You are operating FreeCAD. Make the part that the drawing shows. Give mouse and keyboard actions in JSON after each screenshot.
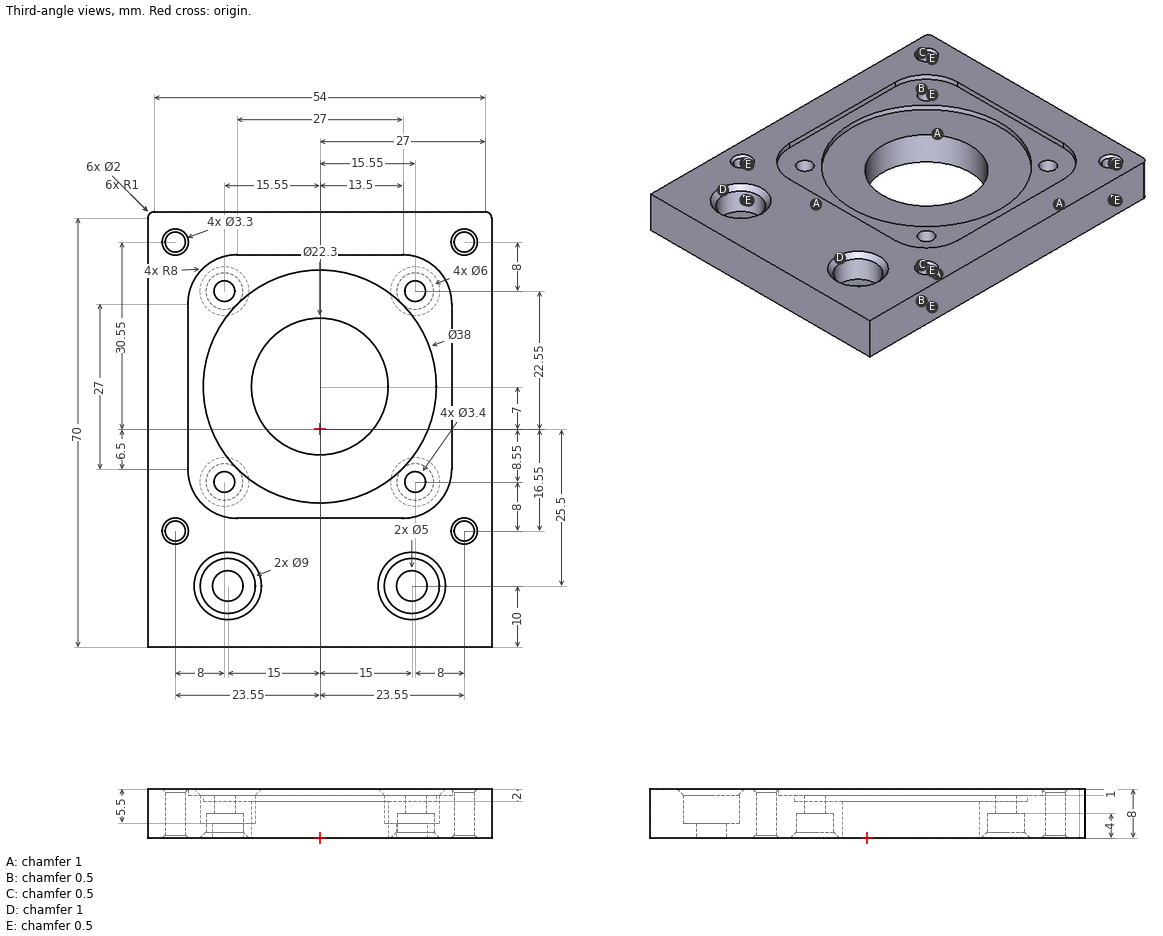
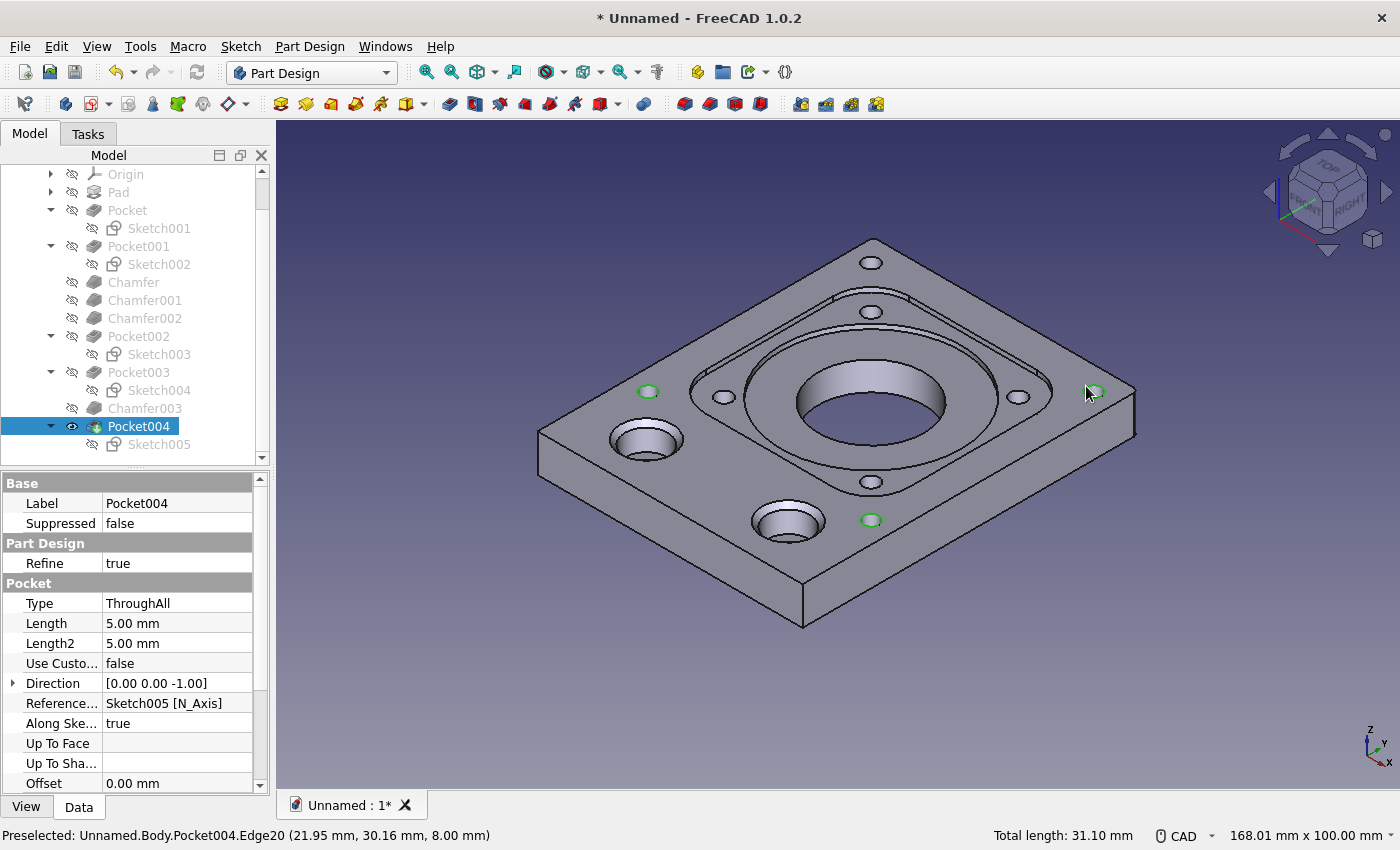
{"action": "left_click", "coordinate": [863, 258], "text": "ctrl"}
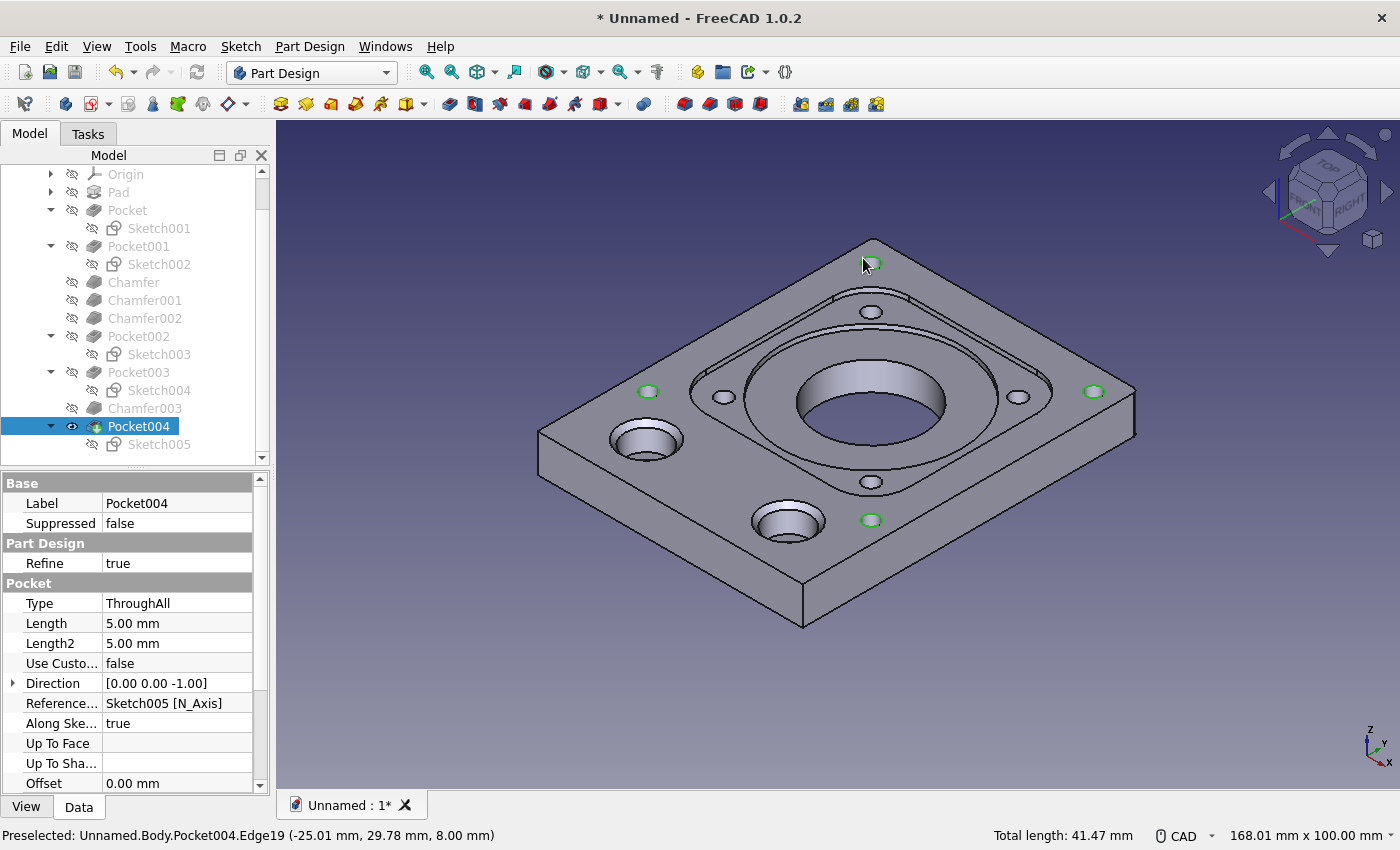
{"action": "key", "text": "2"}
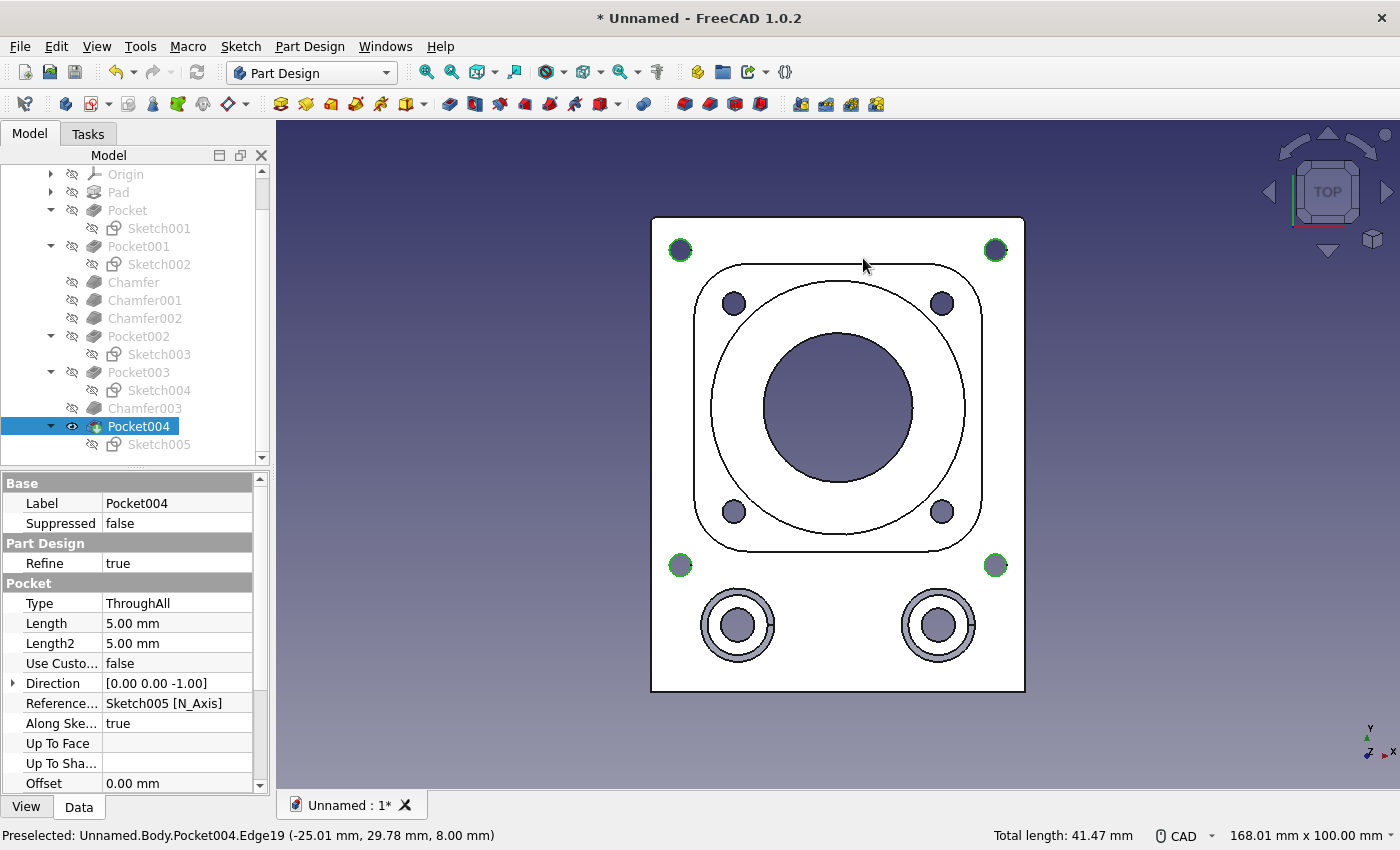
{"action": "key", "text": "0"}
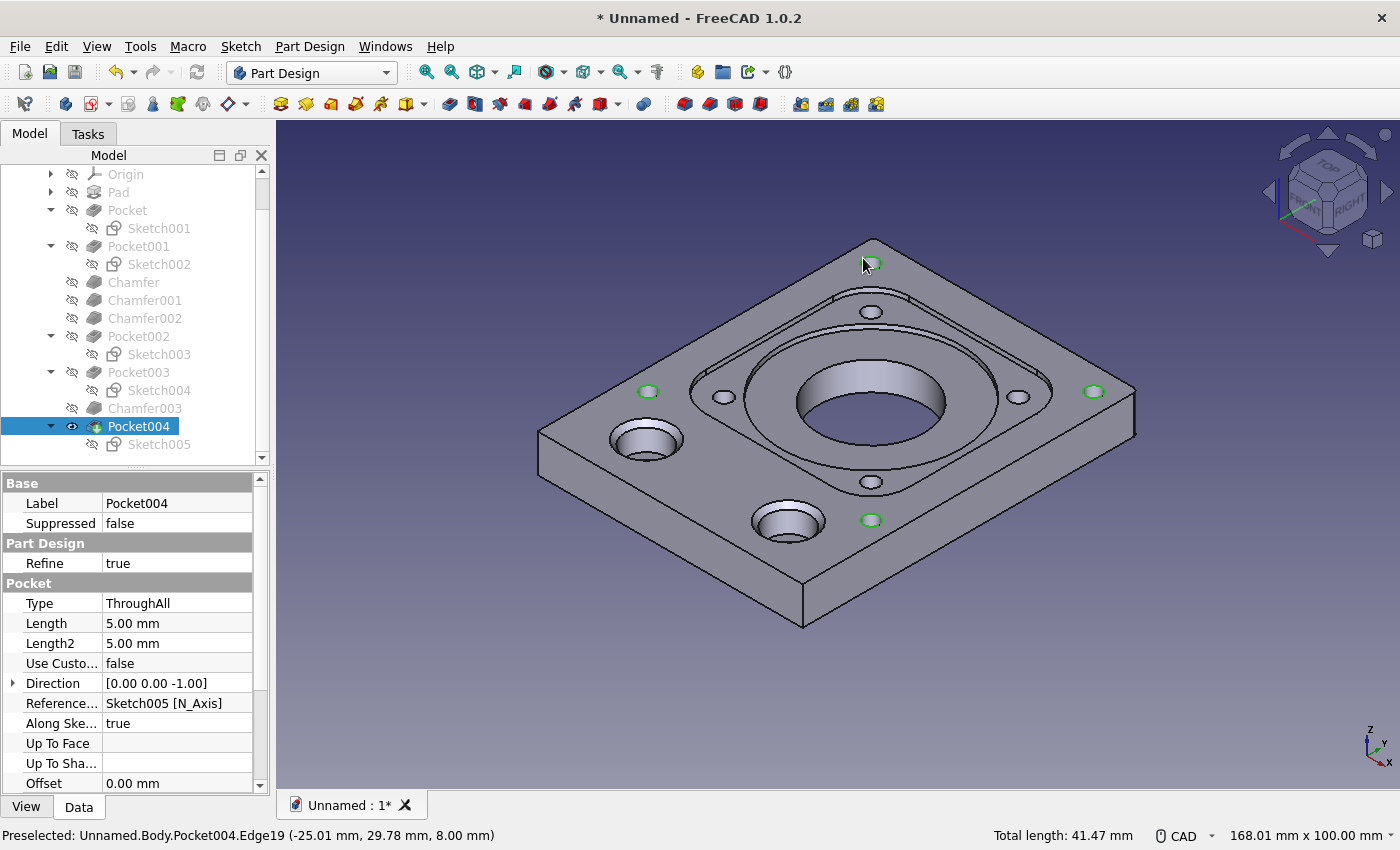
{"action": "key", "text": "1"}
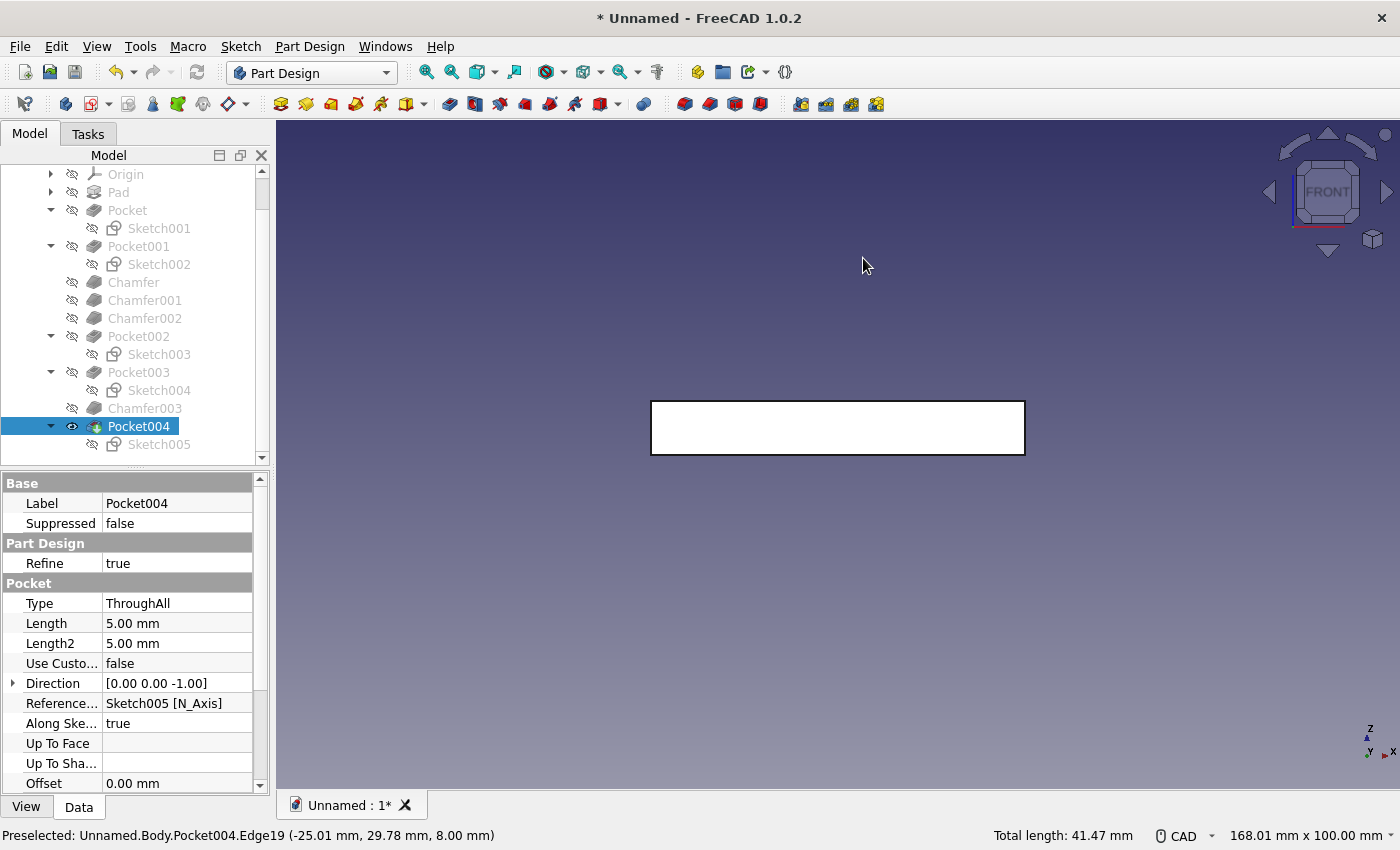
{"action": "key", "text": "v f"}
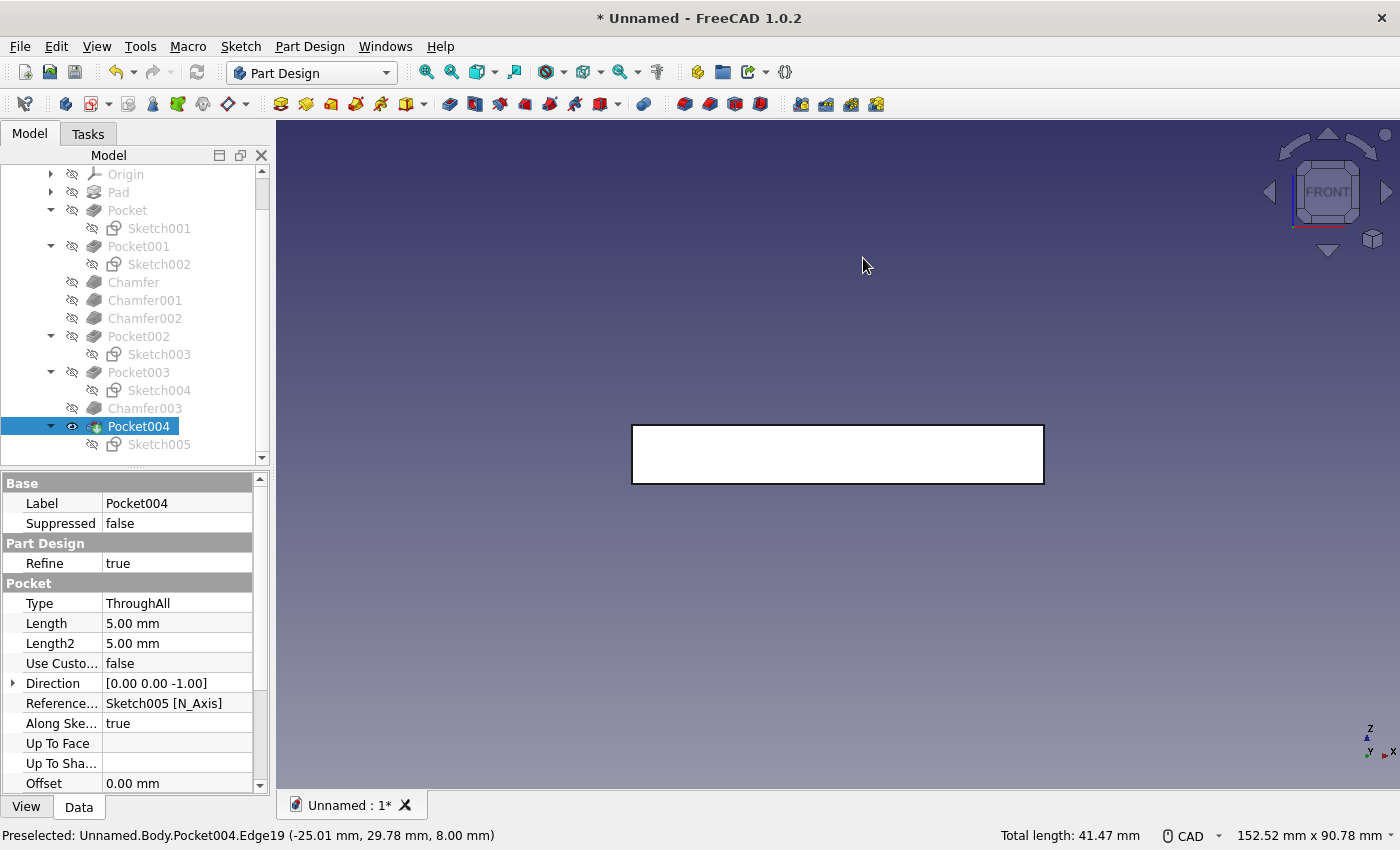
{"action": "key", "text": "3"}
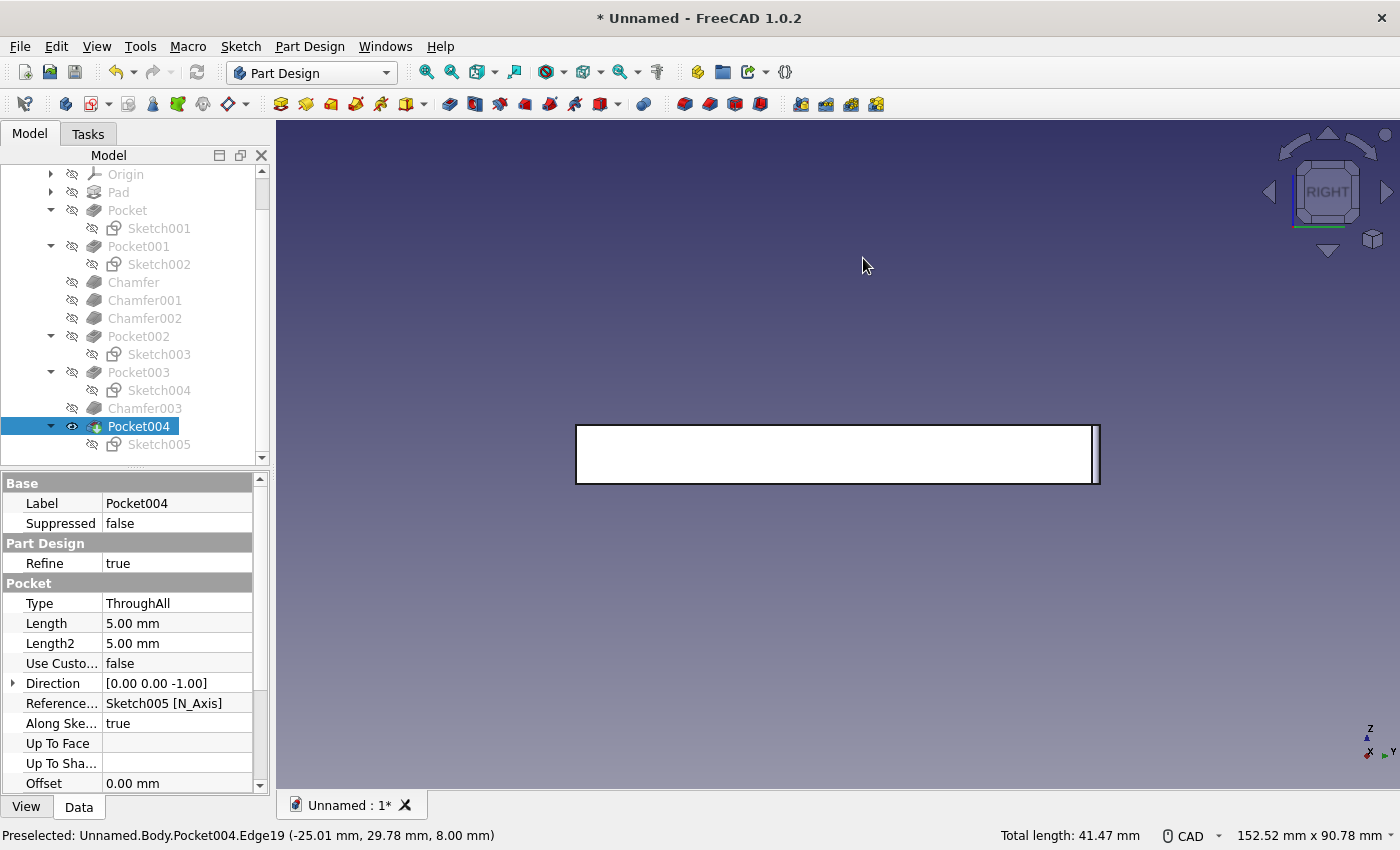
{"action": "key", "text": "5"}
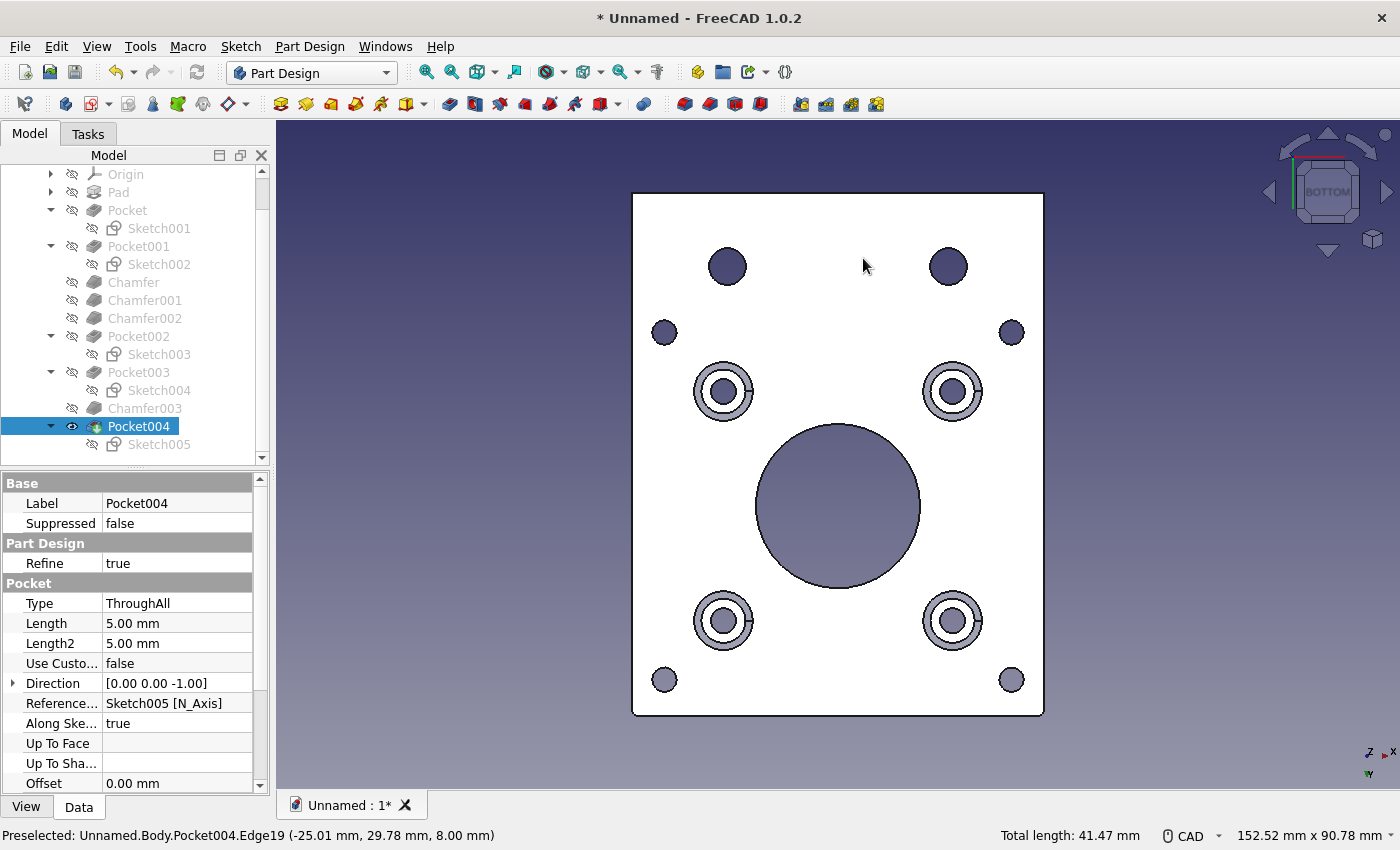
{"action": "left_click", "coordinate": [652, 332], "text": "ctrl"}